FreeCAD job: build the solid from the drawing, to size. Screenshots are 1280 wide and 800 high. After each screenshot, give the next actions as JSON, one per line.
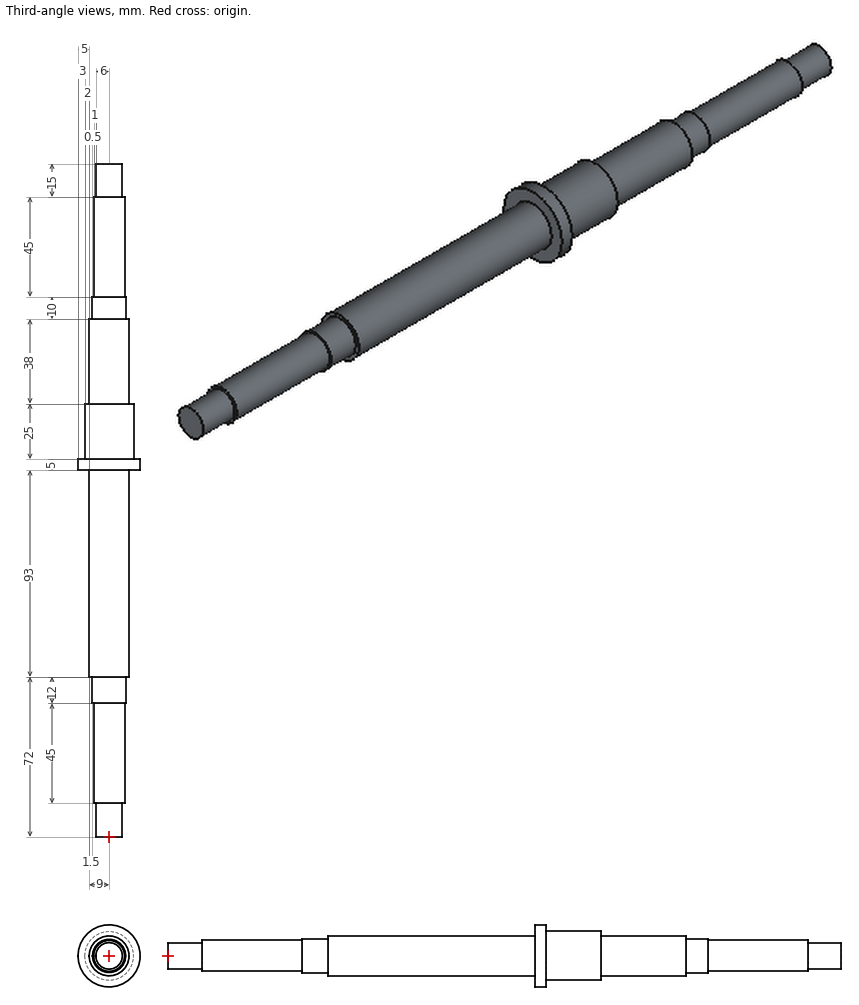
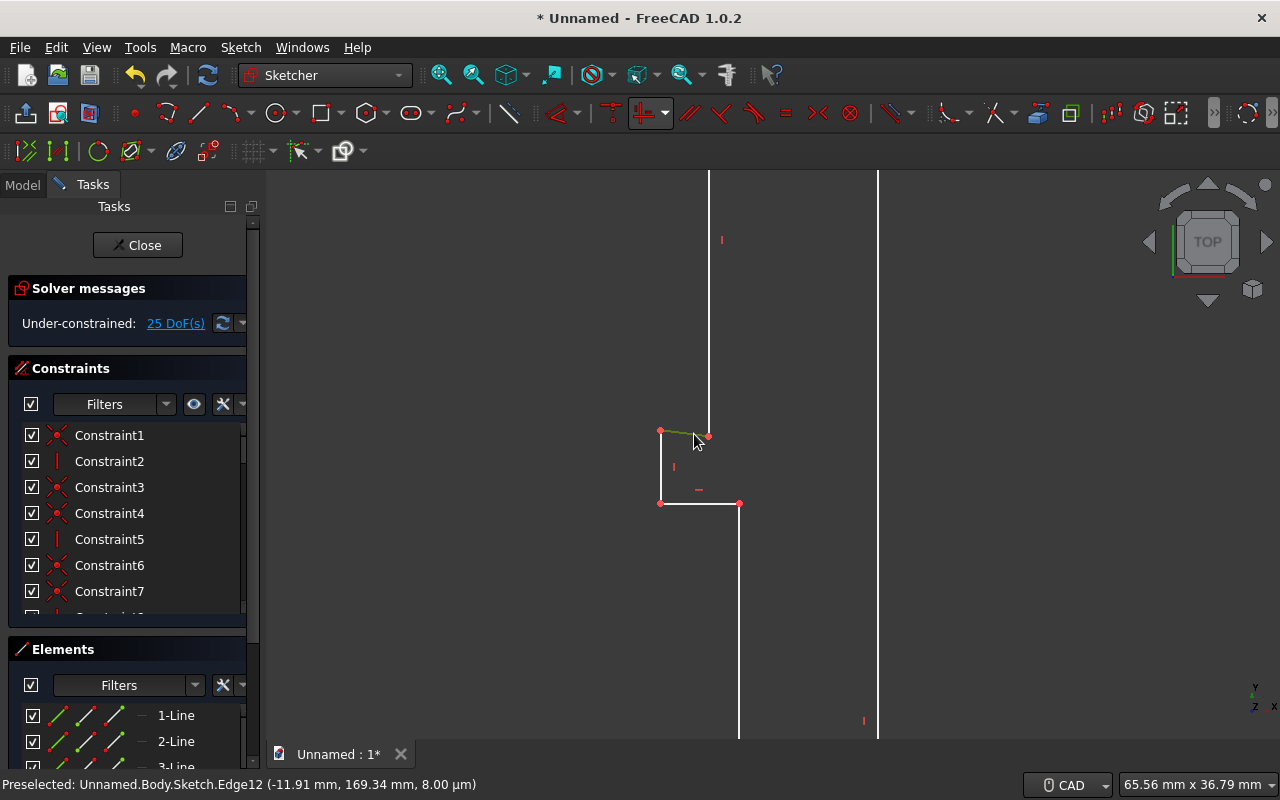
{"action": "key", "text": "h"}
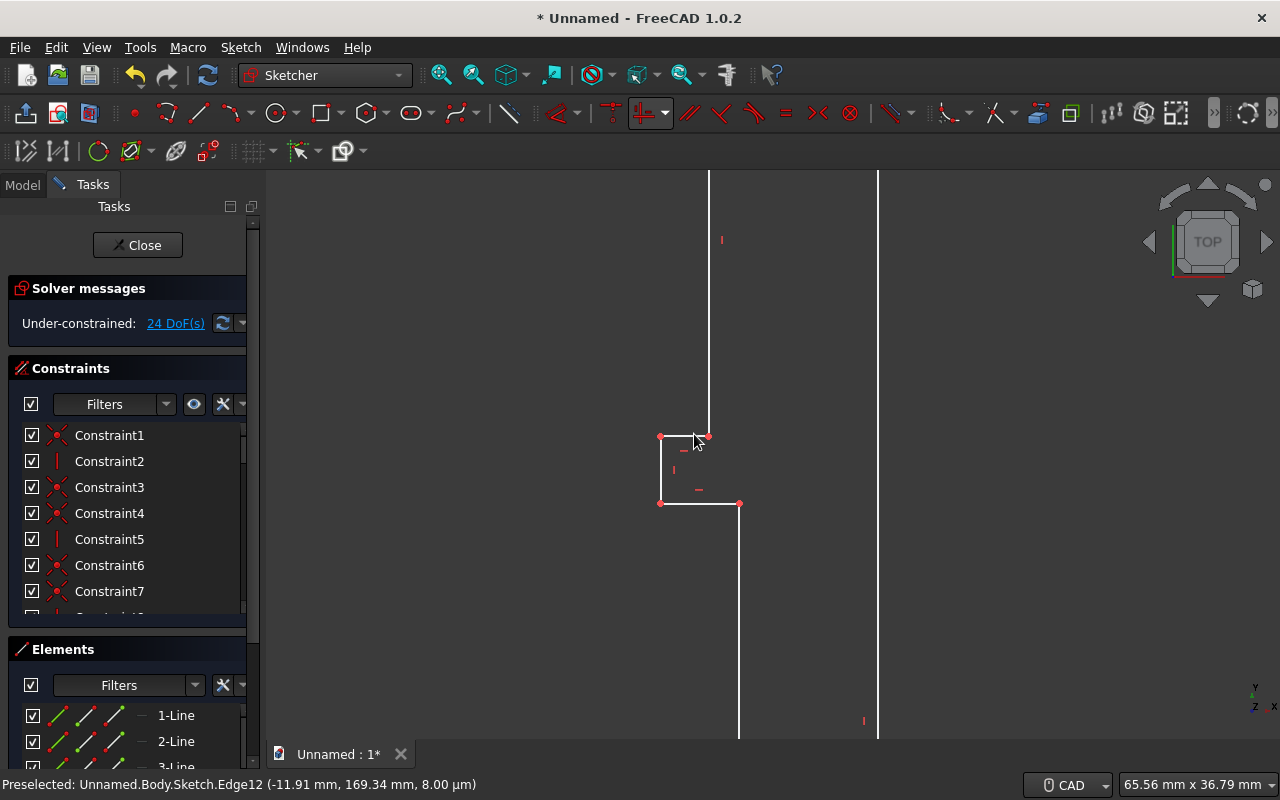
{"action": "scroll", "coordinate": [699, 434], "scroll_direction": "down", "scroll_amount": 13}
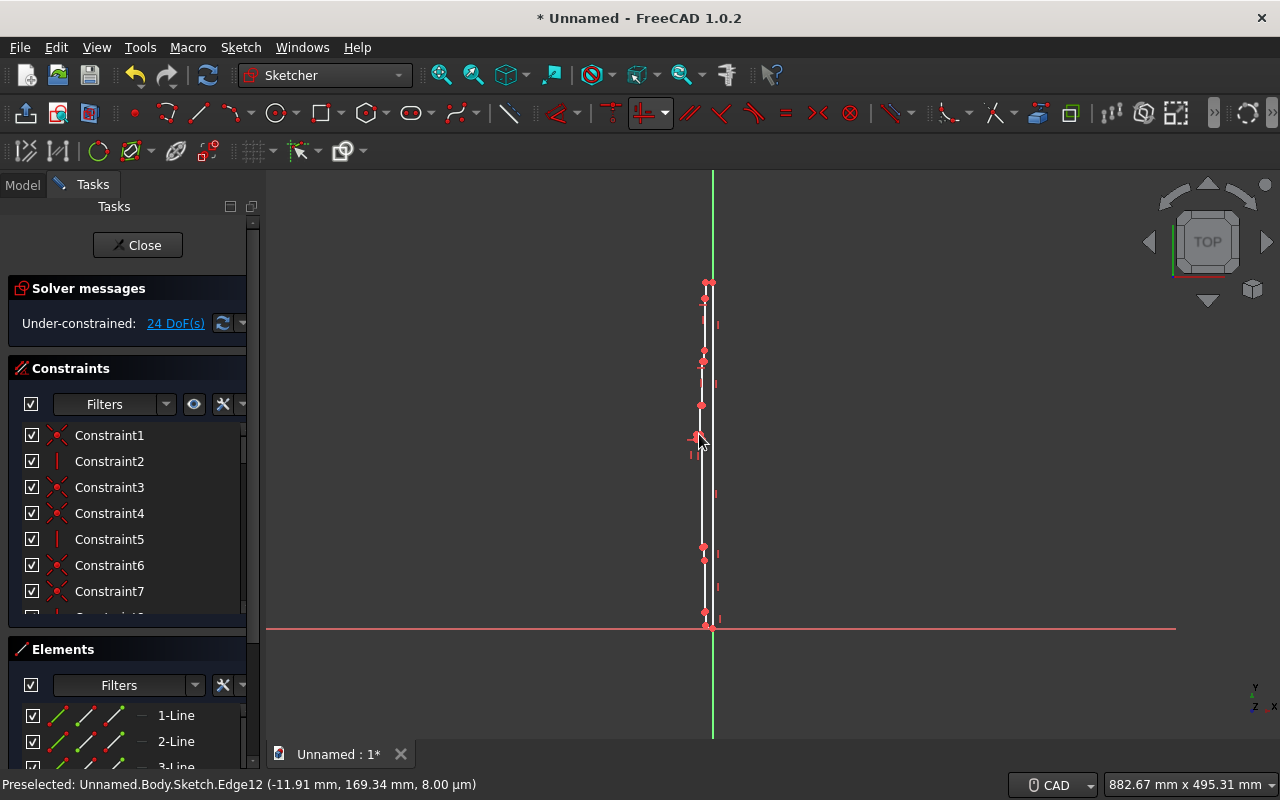
{"action": "scroll", "coordinate": [703, 547], "scroll_direction": "up", "scroll_amount": 14}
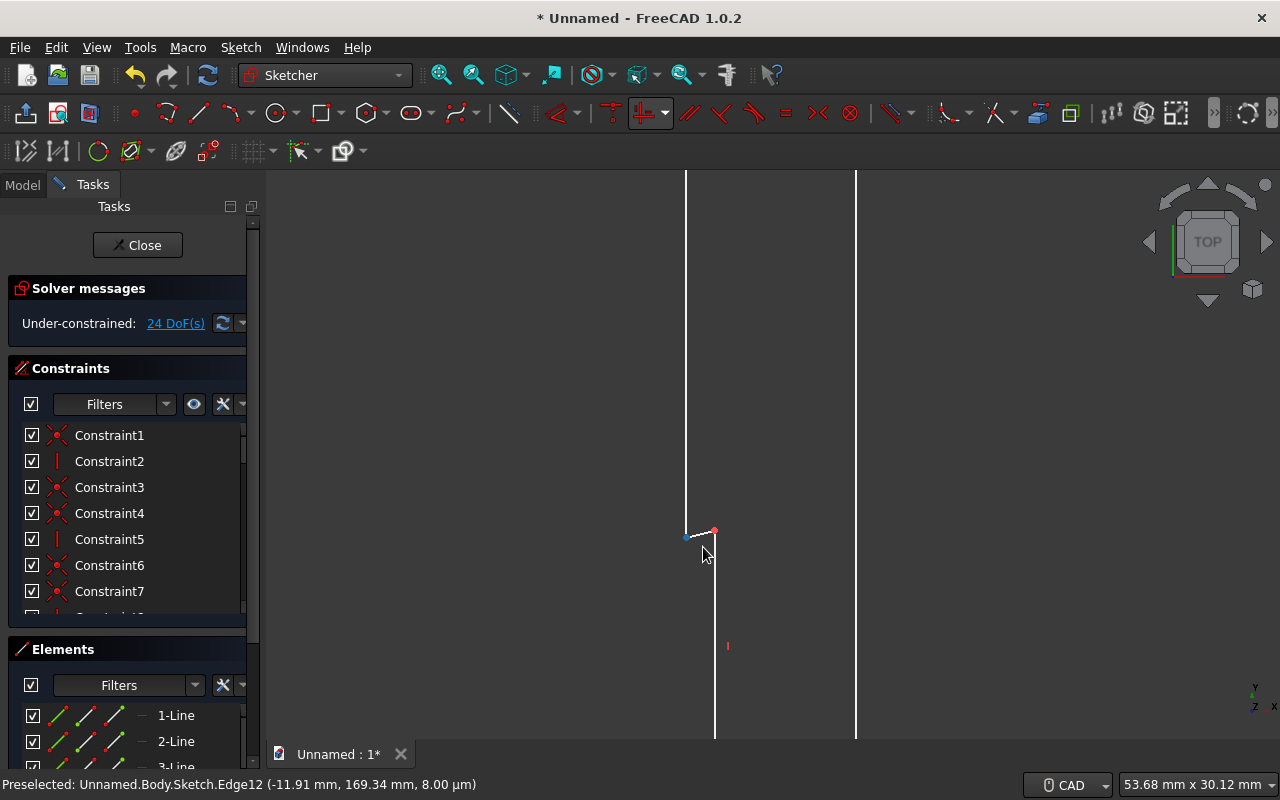
{"action": "left_click", "coordinate": [698, 535]}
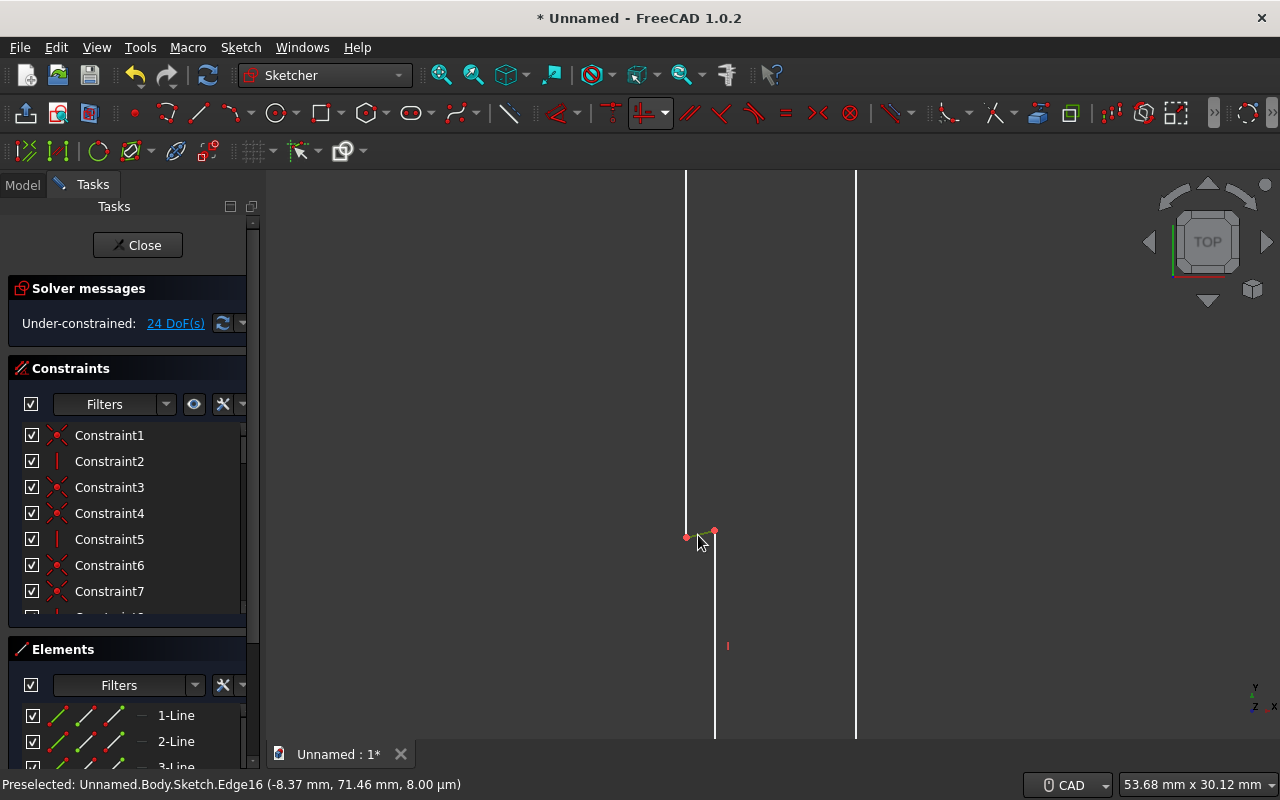
{"action": "left_click", "coordinate": [668, 114]}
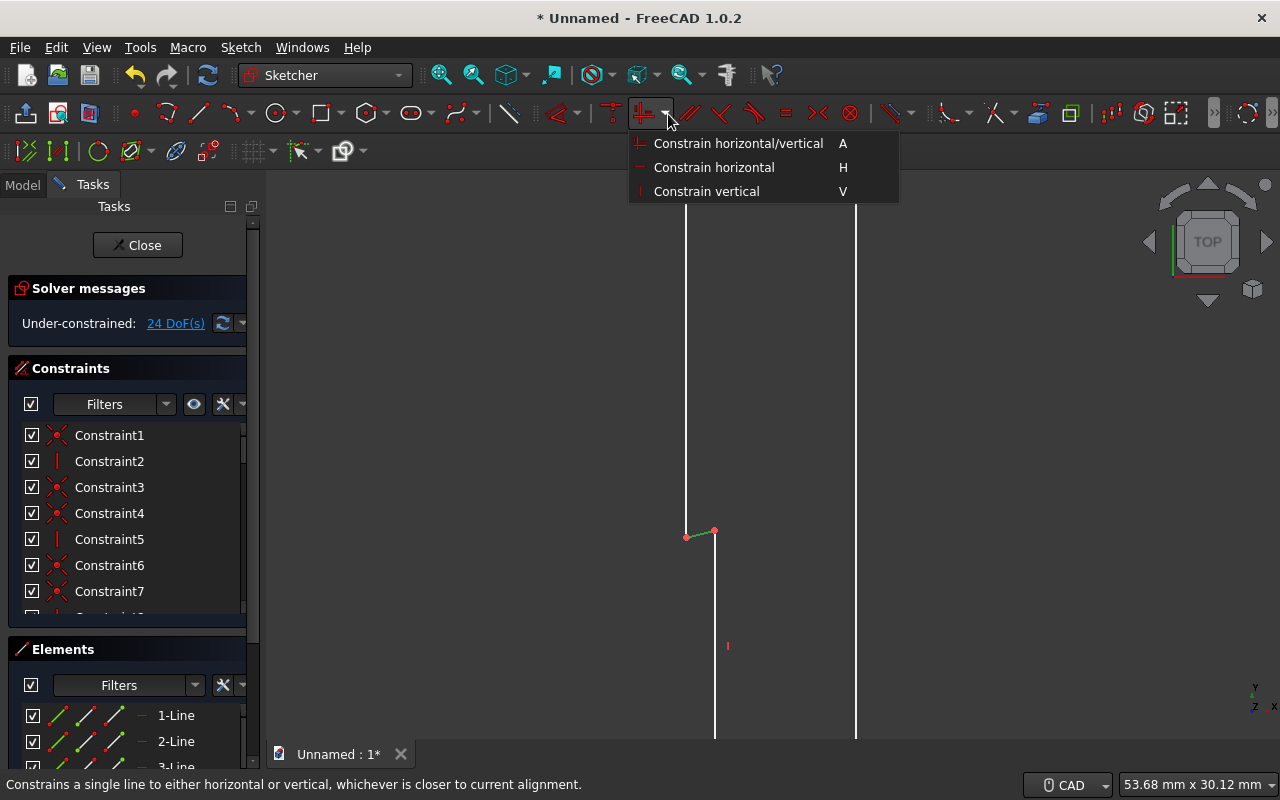
{"action": "left_click", "coordinate": [764, 167]}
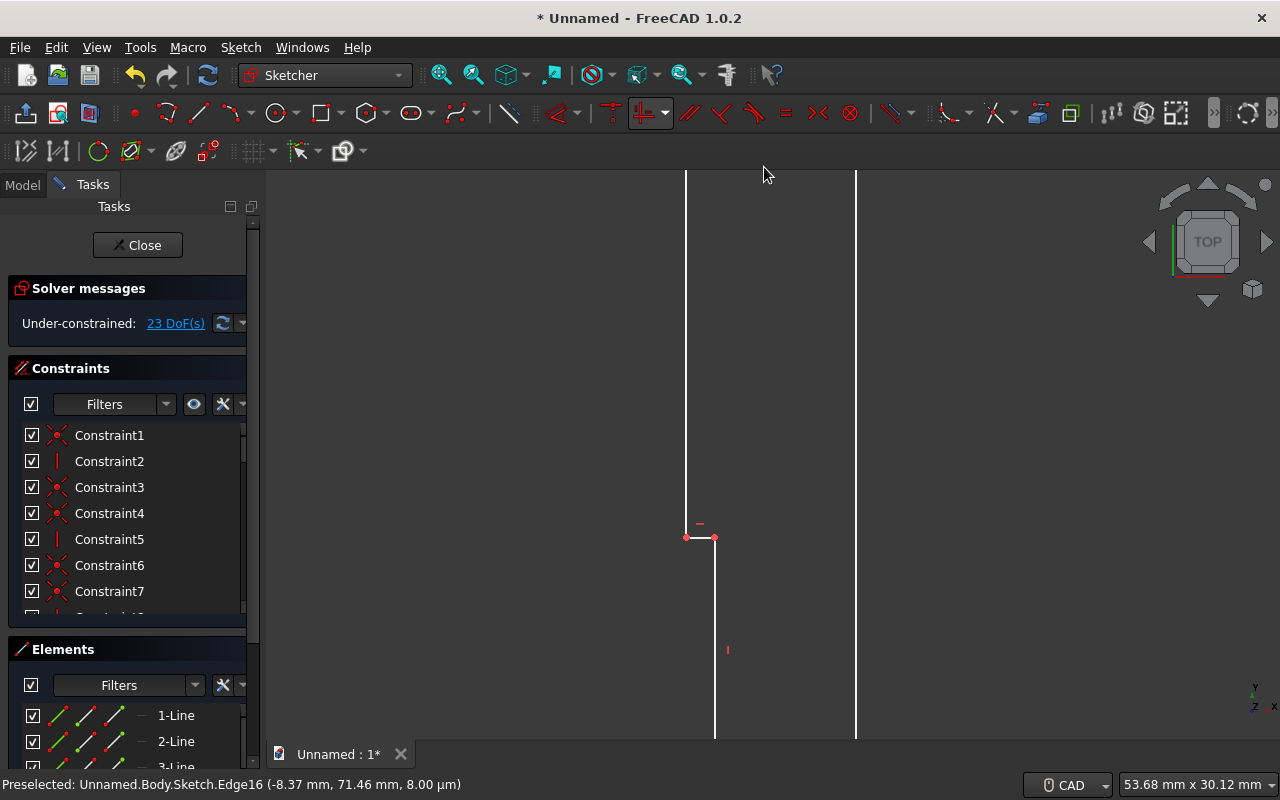
{"action": "scroll", "coordinate": [703, 547], "scroll_direction": "down", "scroll_amount": 14}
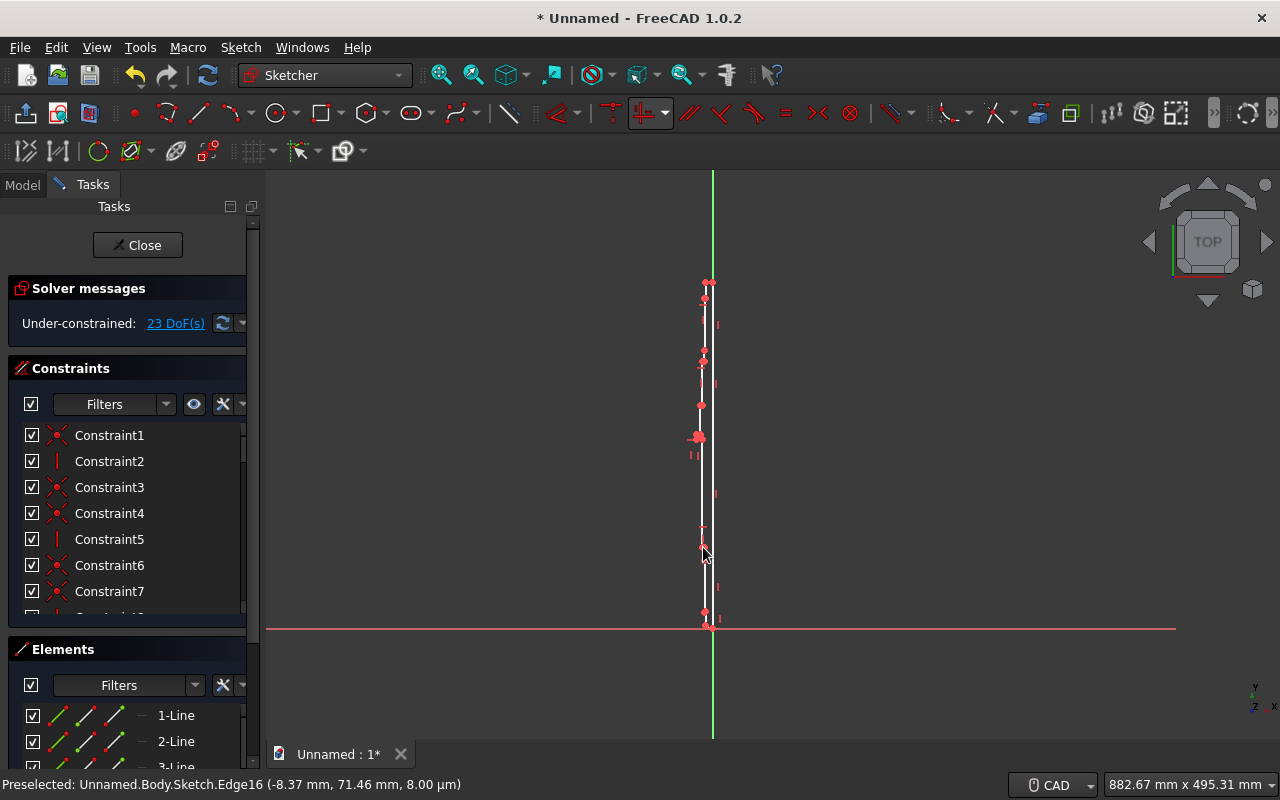
{"action": "scroll", "coordinate": [704, 560], "scroll_direction": "up", "scroll_amount": 14}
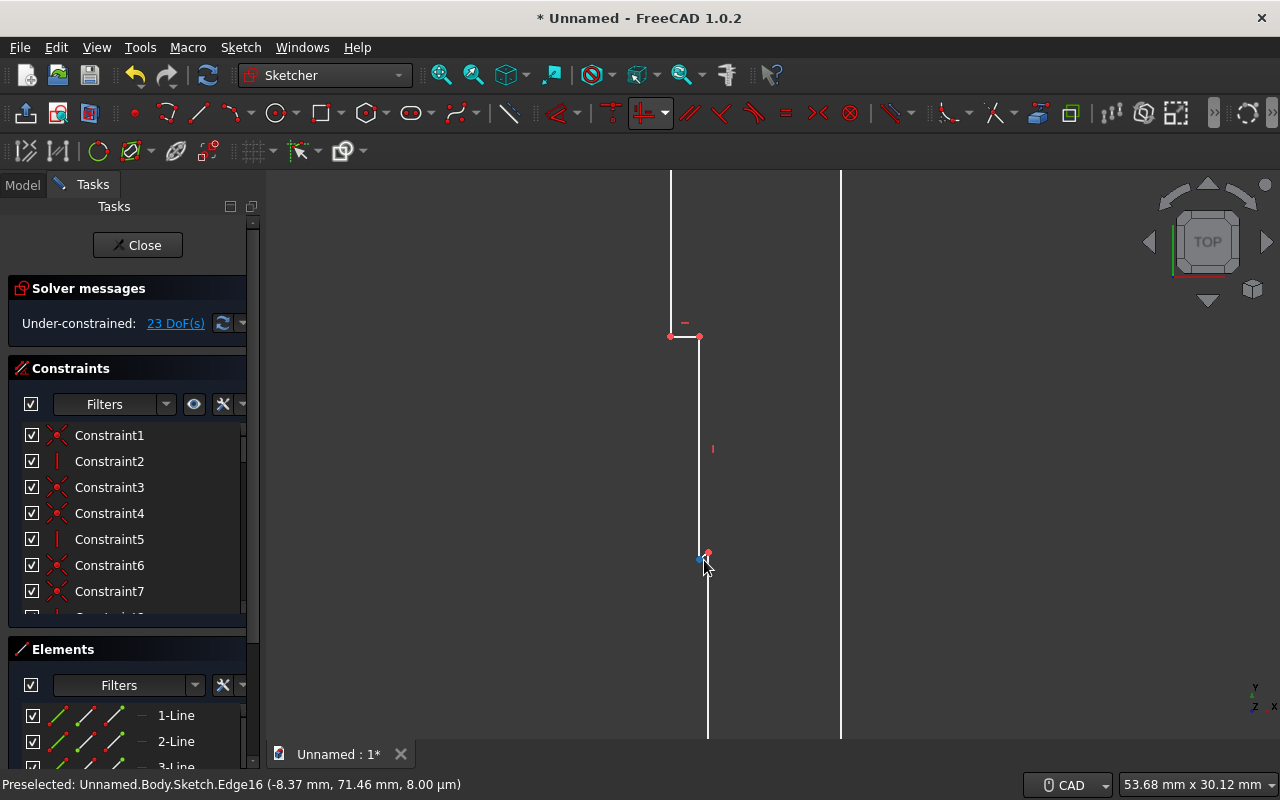
{"action": "left_click", "coordinate": [704, 556]}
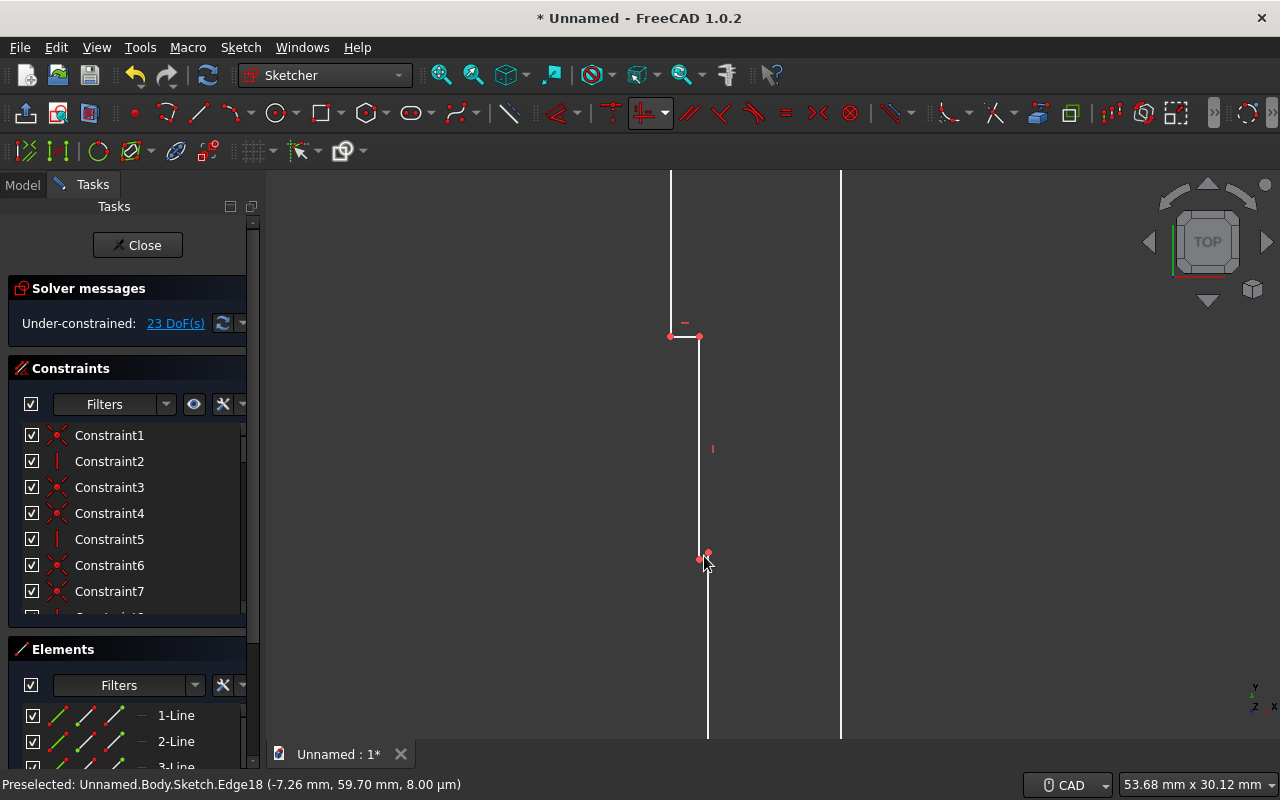
{"action": "key", "text": "h"}